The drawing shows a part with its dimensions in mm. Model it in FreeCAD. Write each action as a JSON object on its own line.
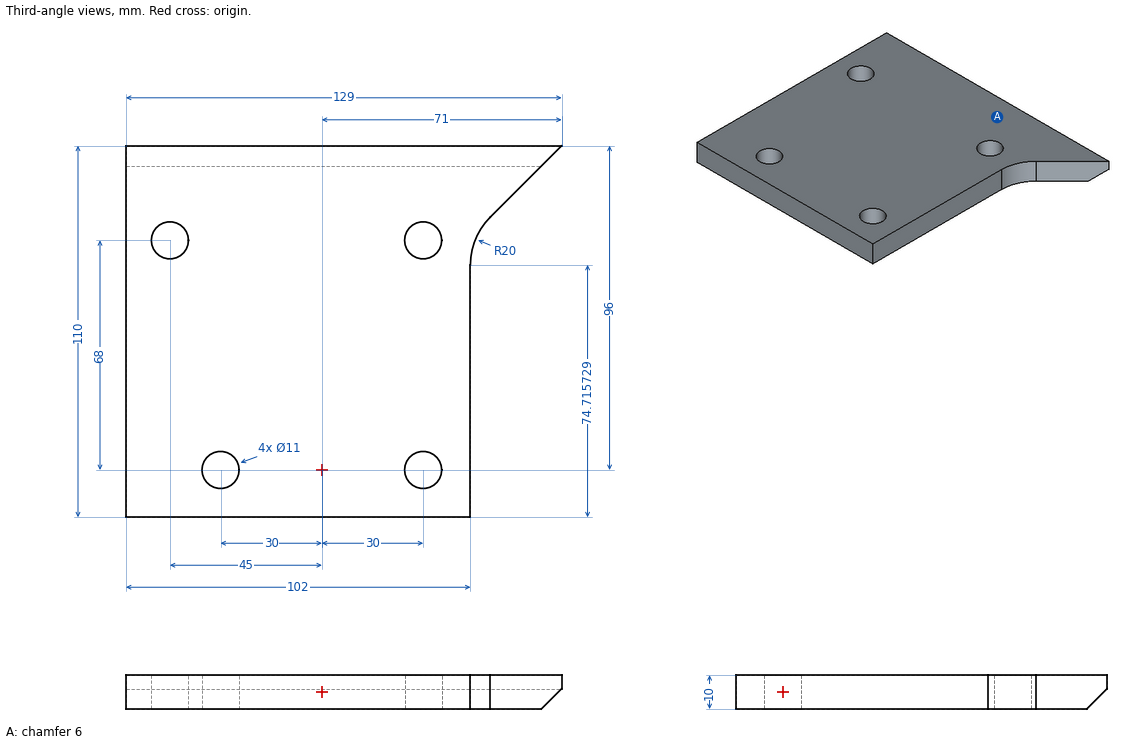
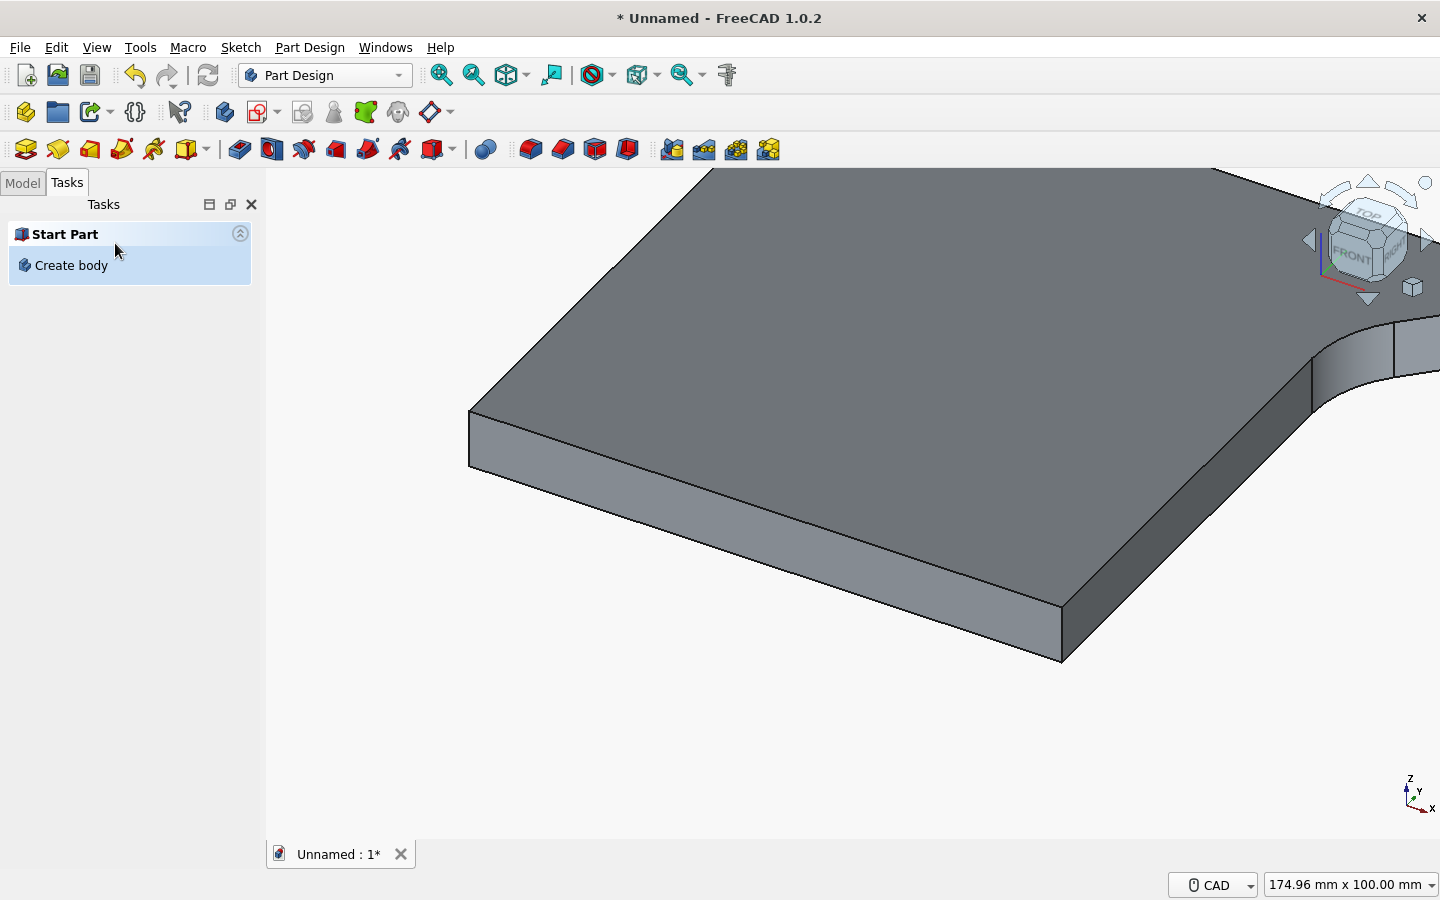
{"action": "left_click", "coordinate": [442, 76]}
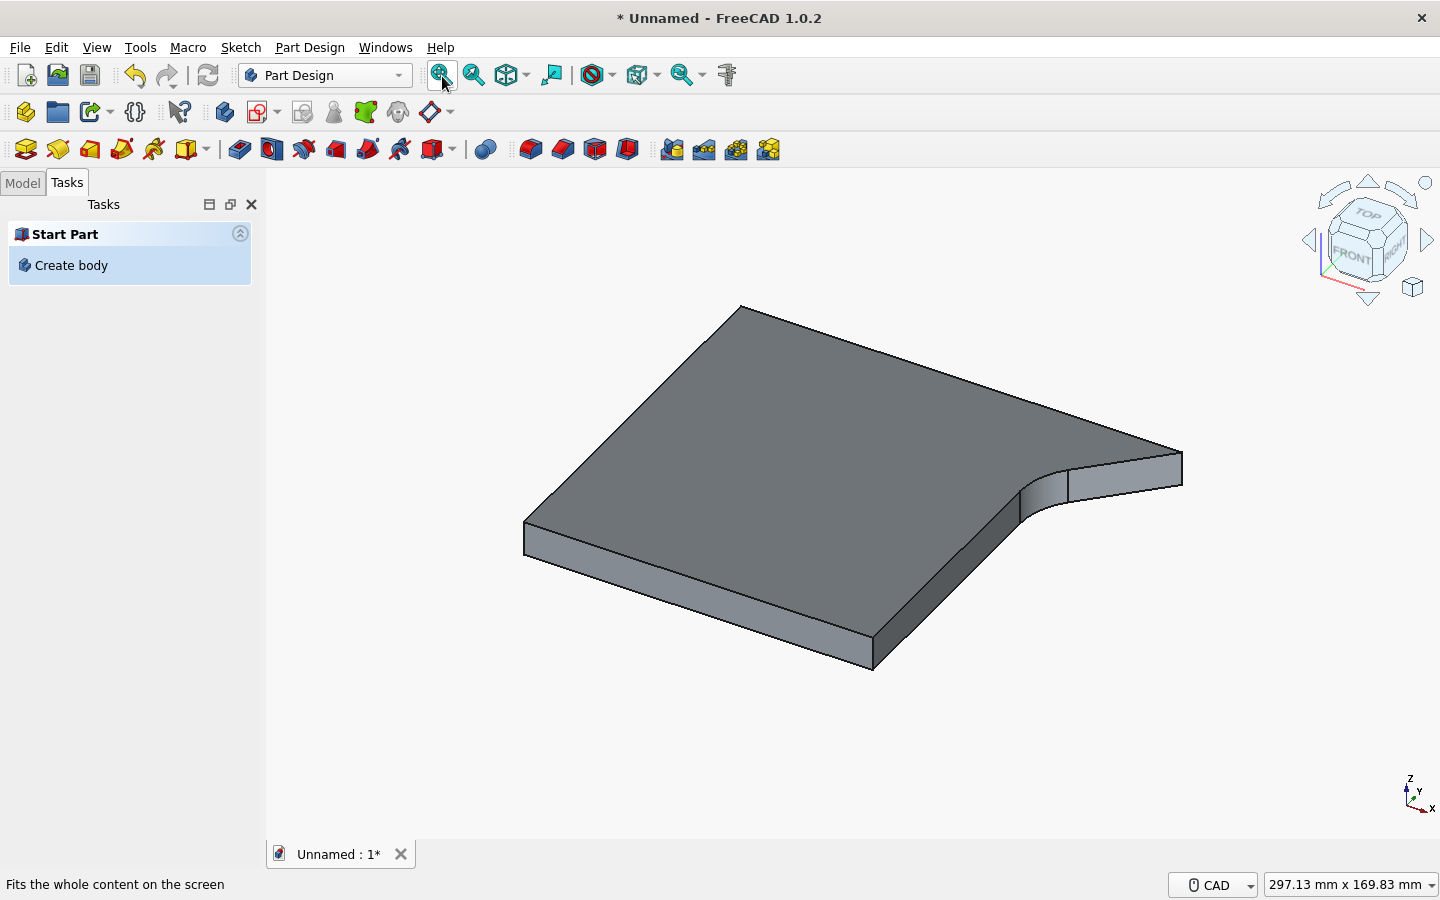
{"action": "left_click", "coordinate": [258, 112]}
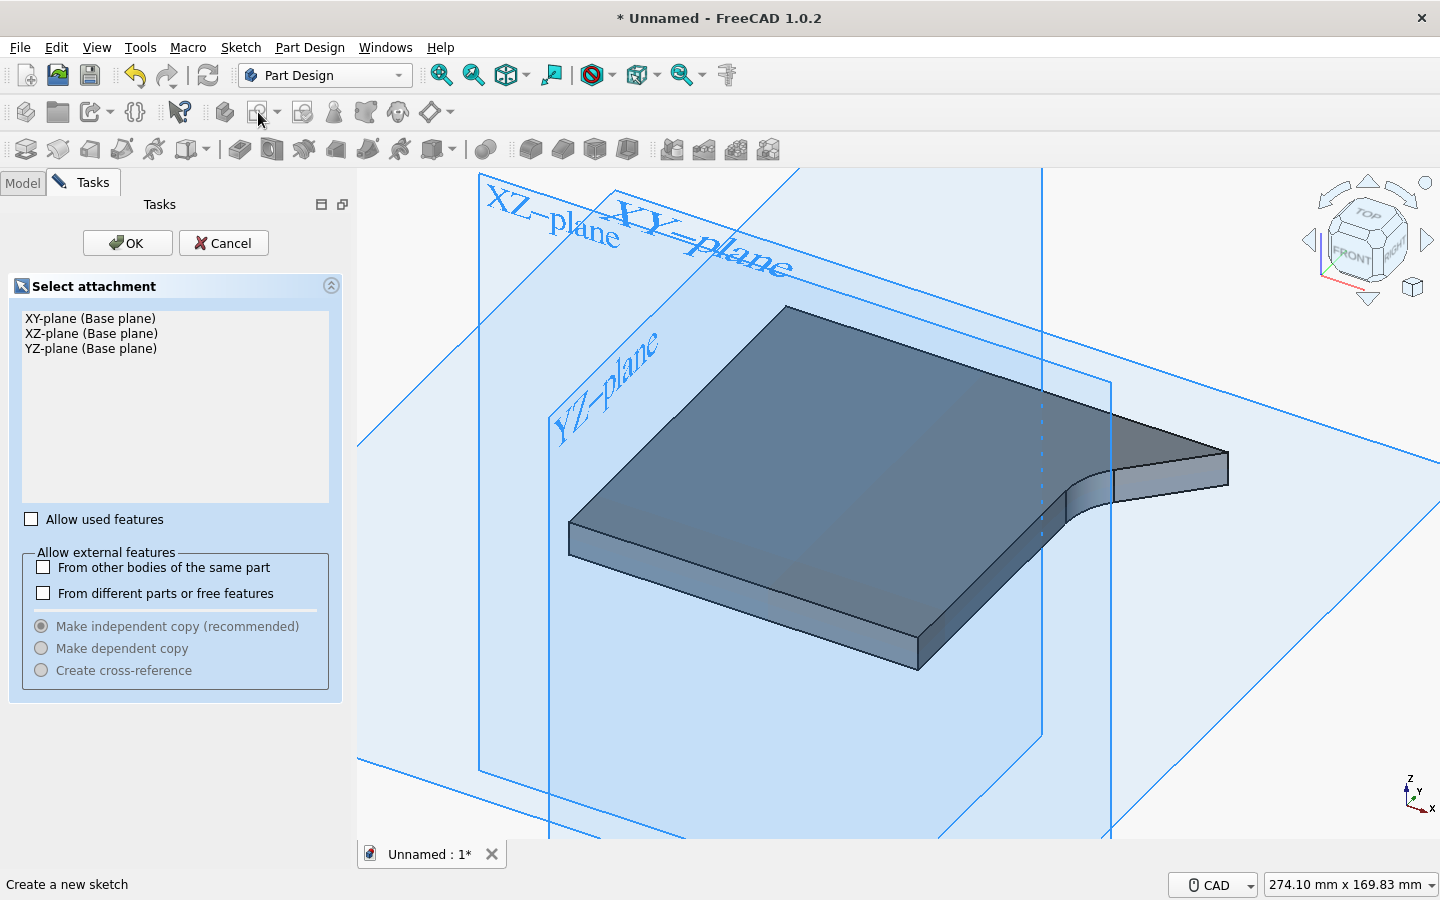
{"action": "left_click", "coordinate": [82, 318]}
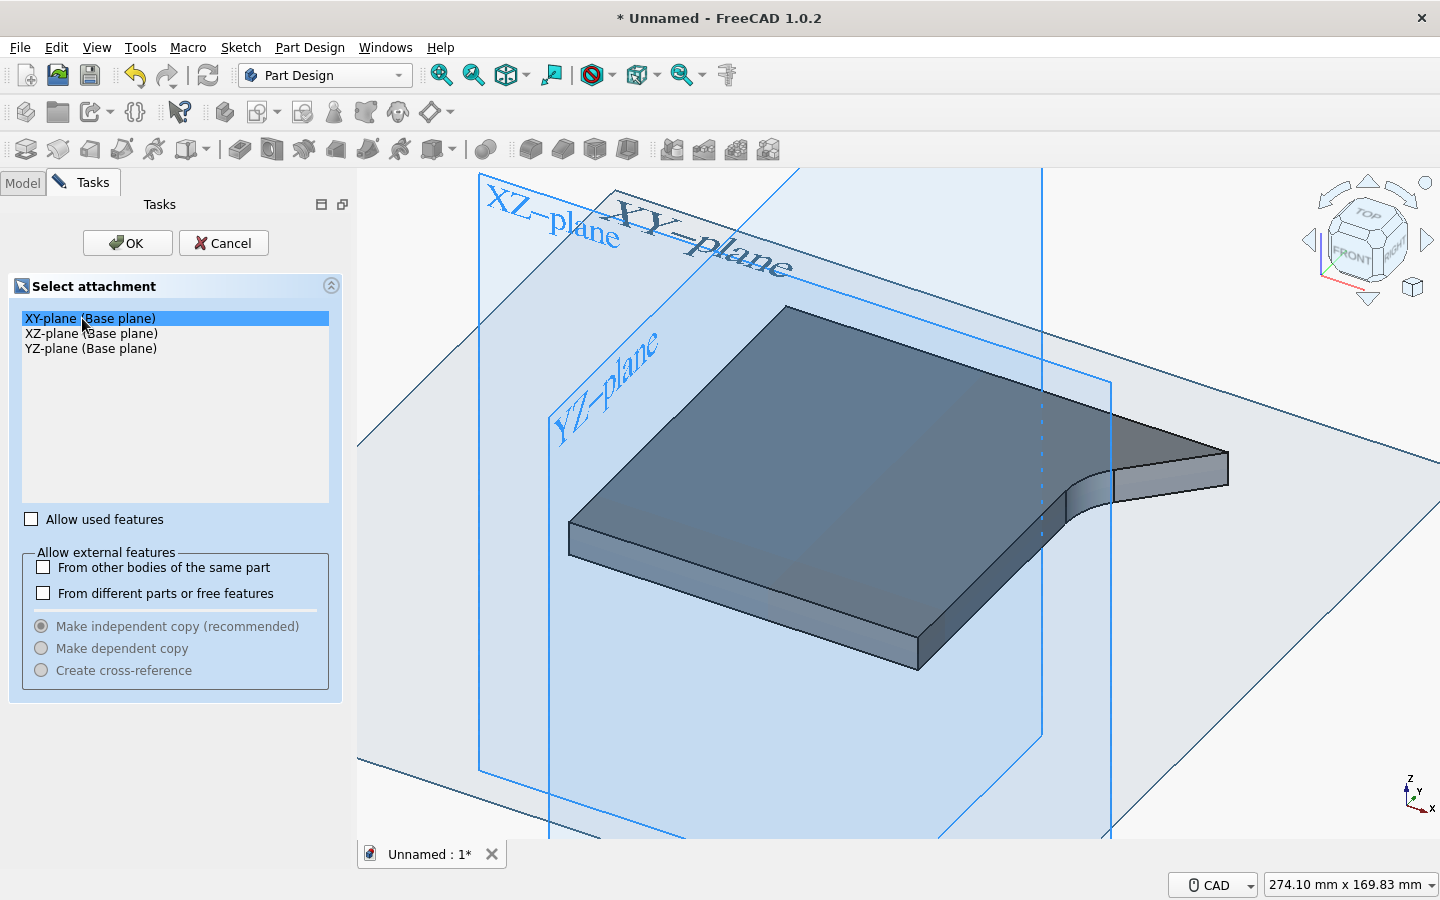
{"action": "left_click", "coordinate": [128, 243]}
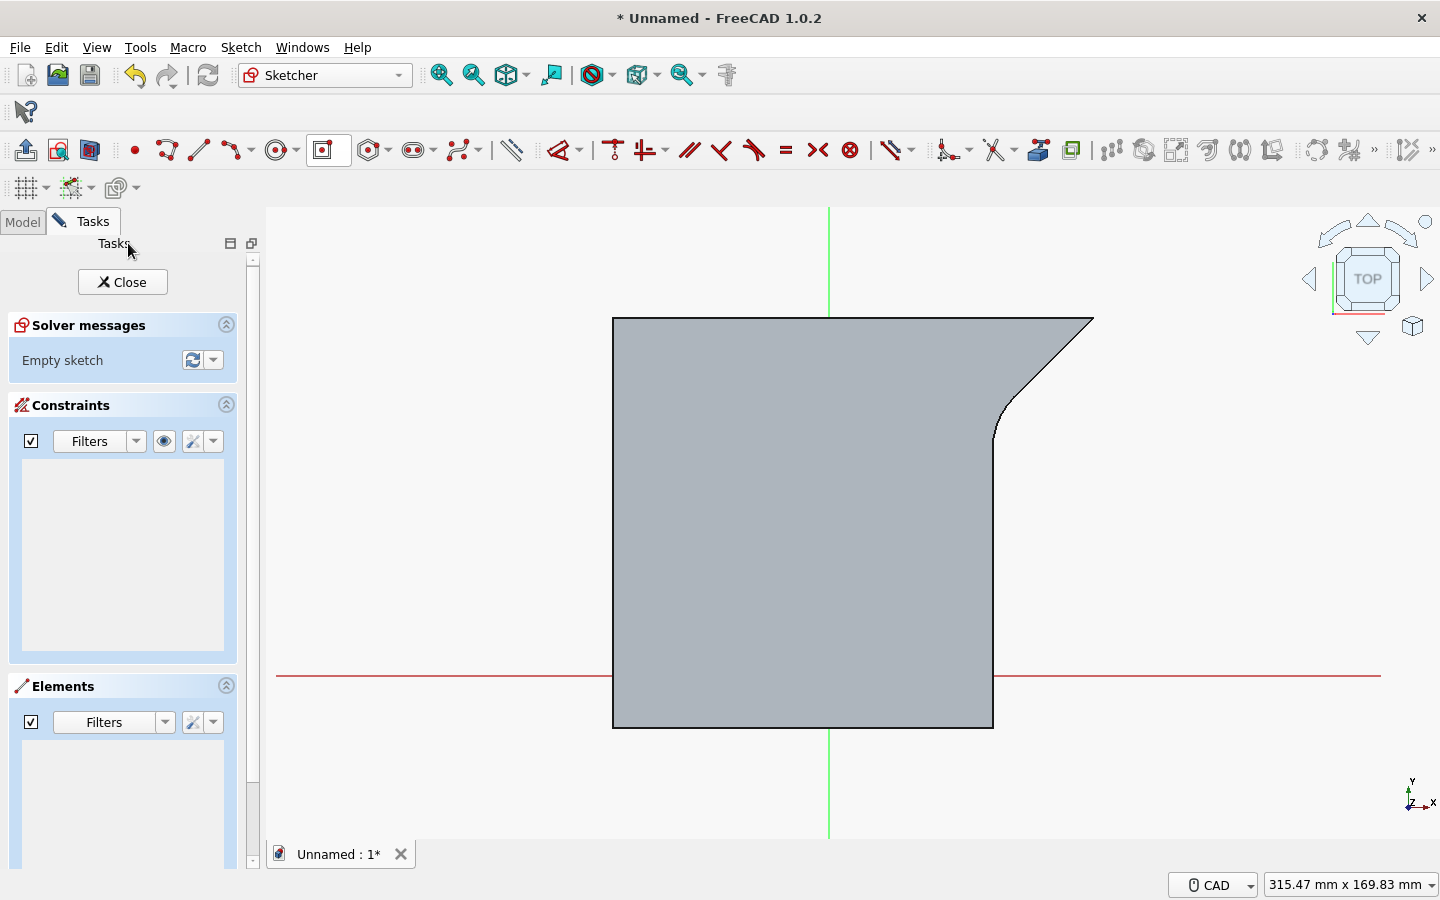
{"action": "left_click", "coordinate": [90, 150]}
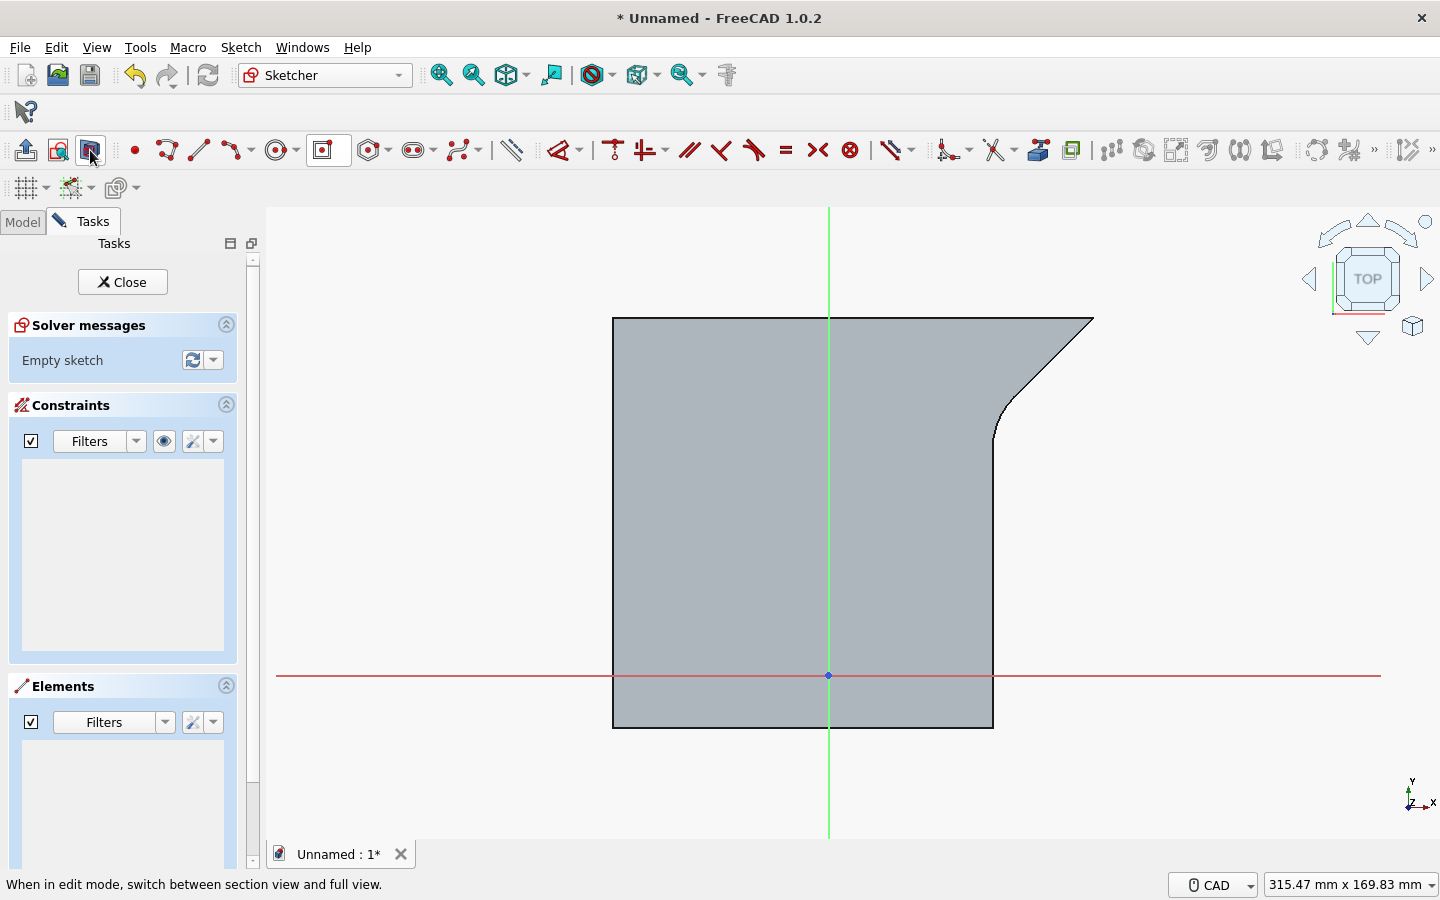
{"action": "scroll", "coordinate": [834, 602], "scroll_direction": "up", "scroll_amount": 2}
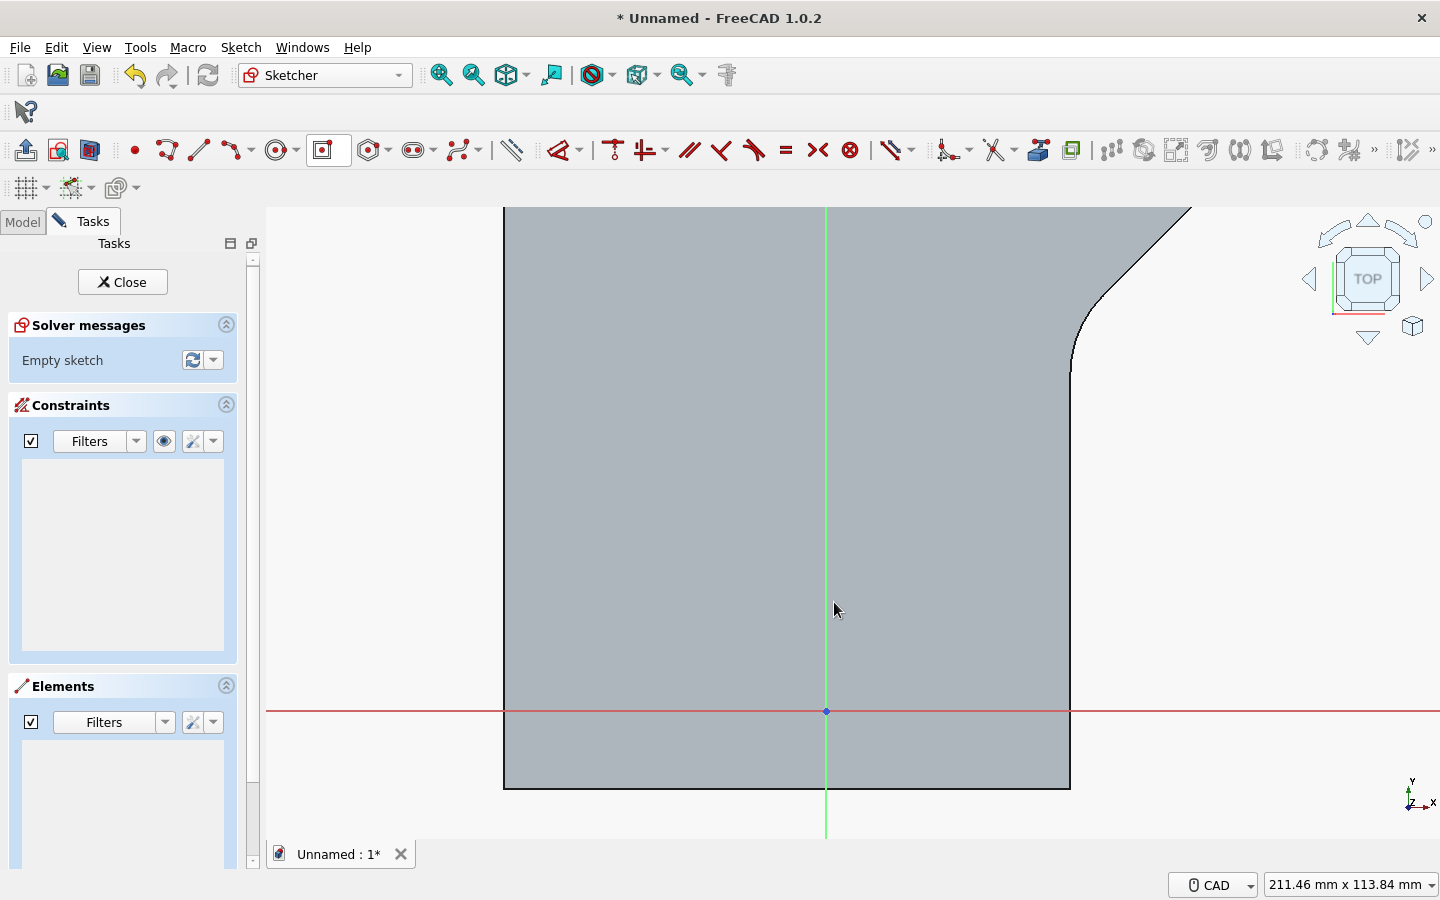
{"action": "left_click", "coordinate": [276, 150]}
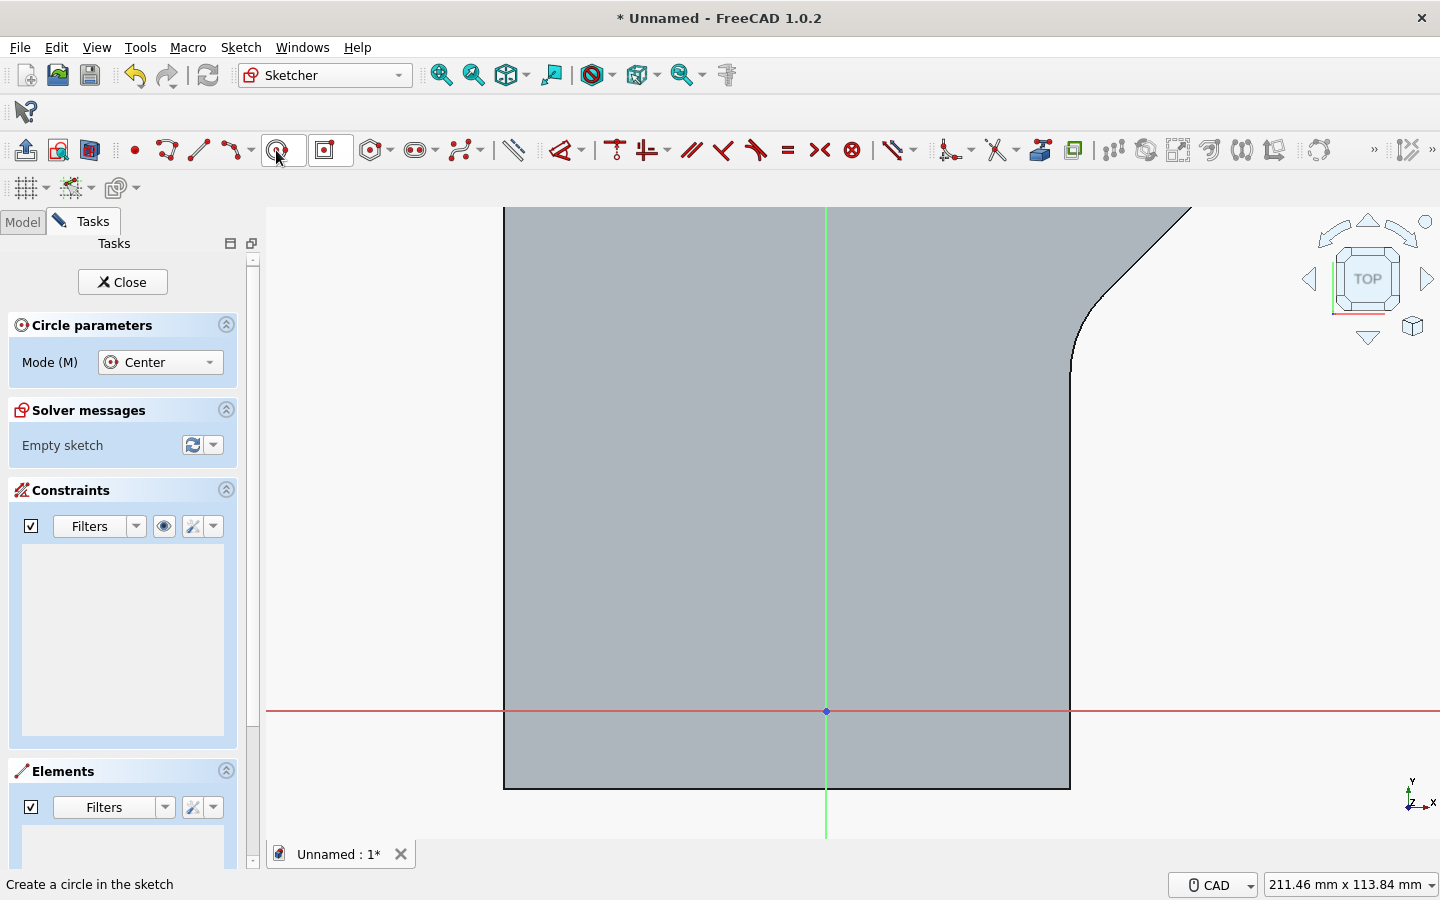
{"action": "left_click", "coordinate": [659, 711]}
{"action": "left_click", "coordinate": [681, 690]}